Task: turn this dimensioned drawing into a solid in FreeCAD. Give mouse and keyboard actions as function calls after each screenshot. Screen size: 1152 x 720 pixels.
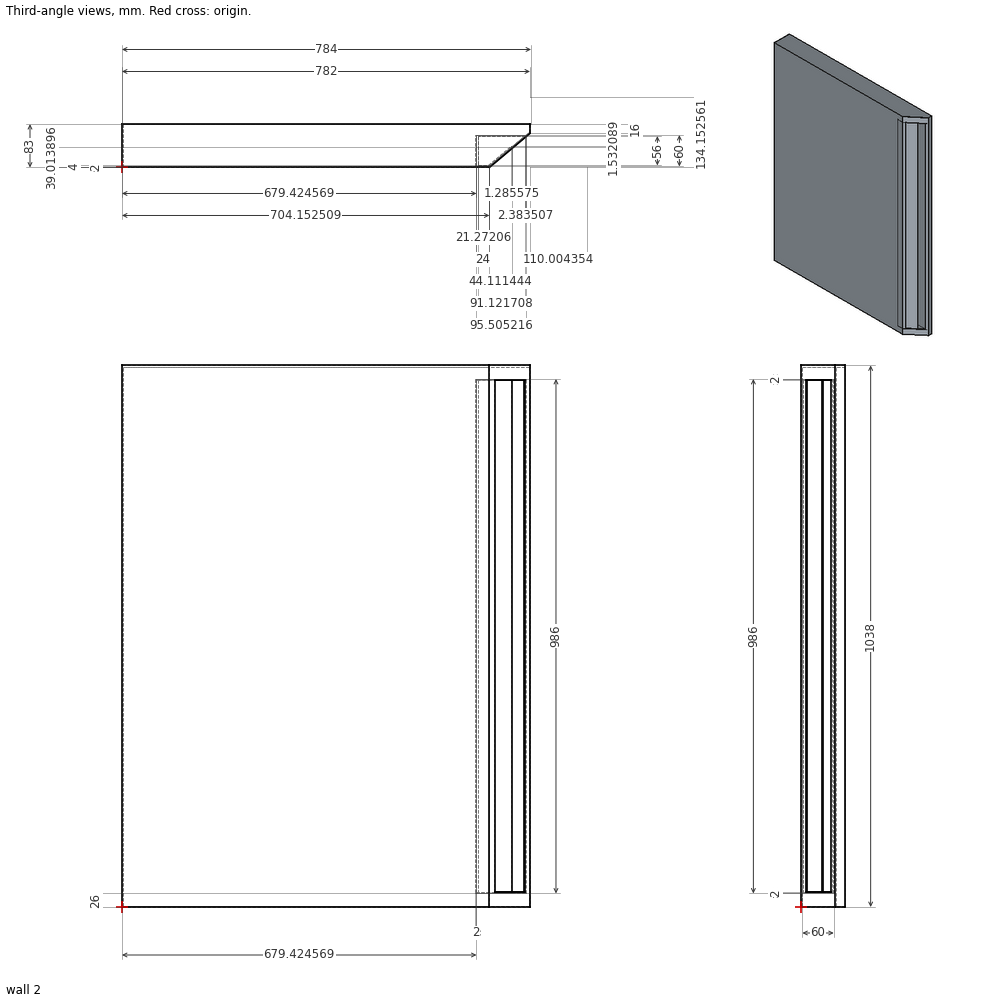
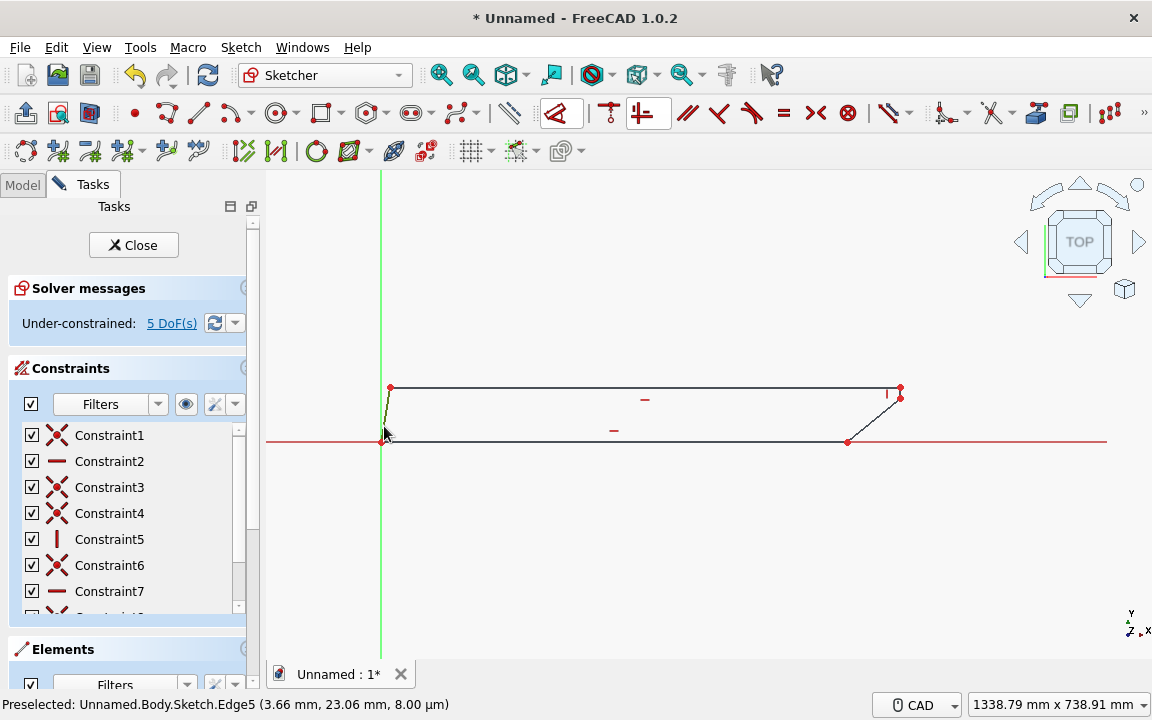
click(666, 114)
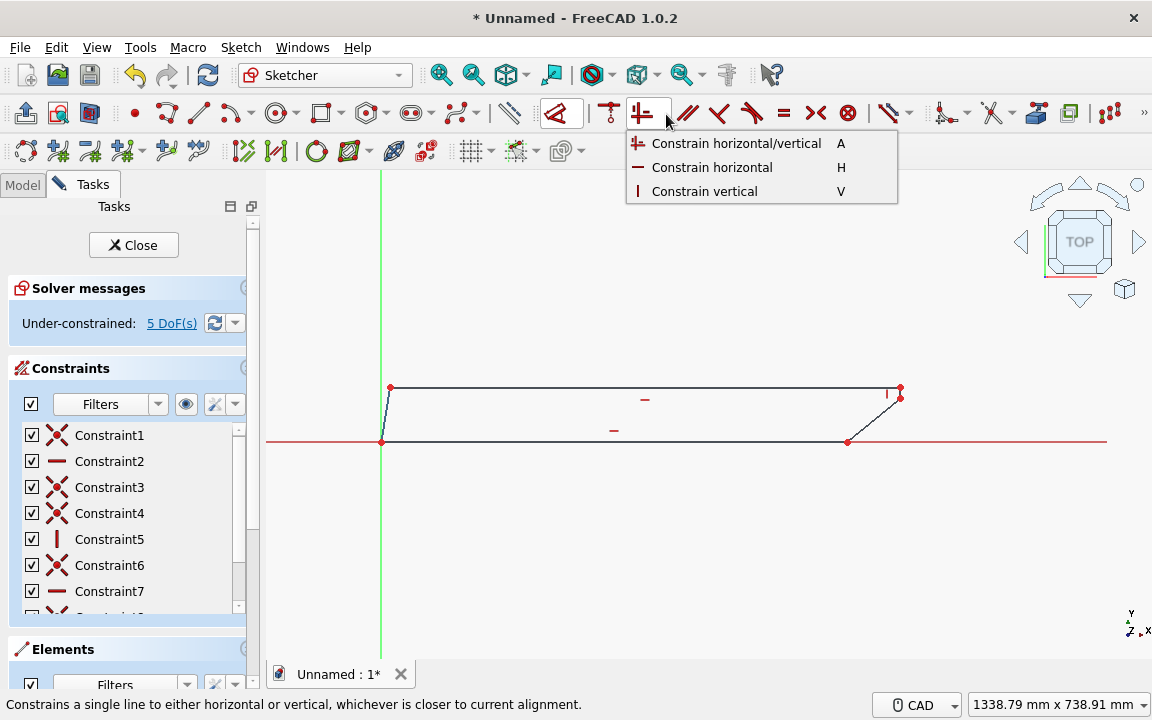
click(762, 191)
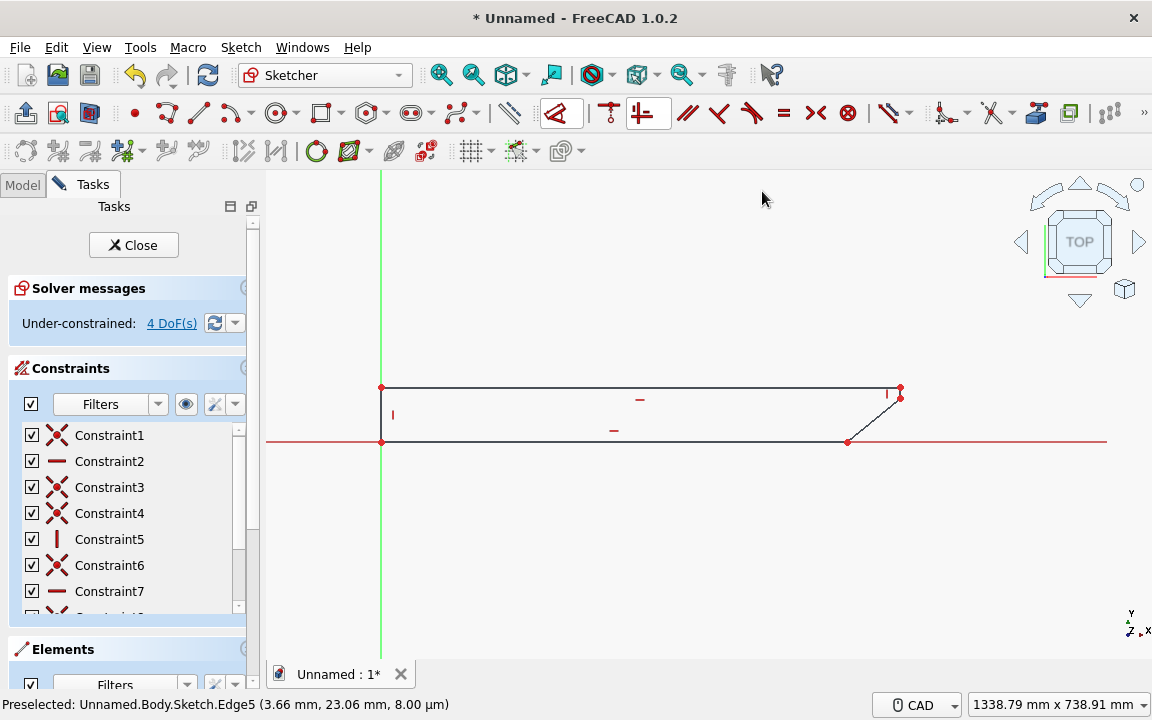
click(556, 114)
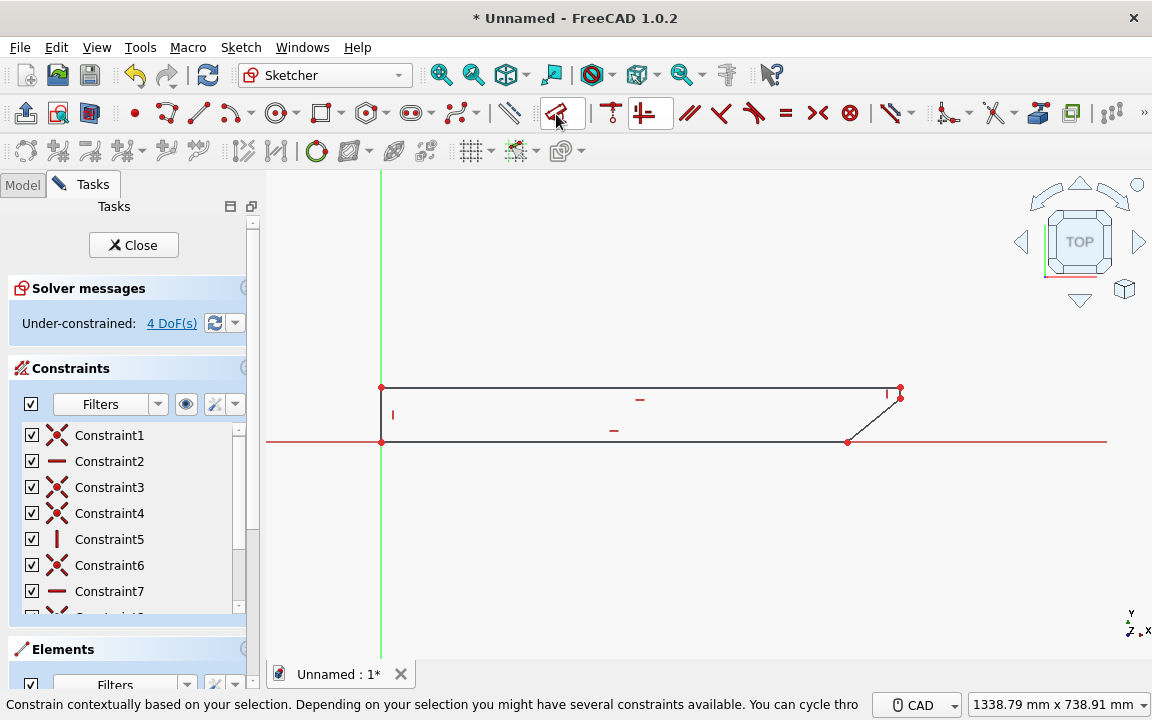
scroll(900, 393, up, 7)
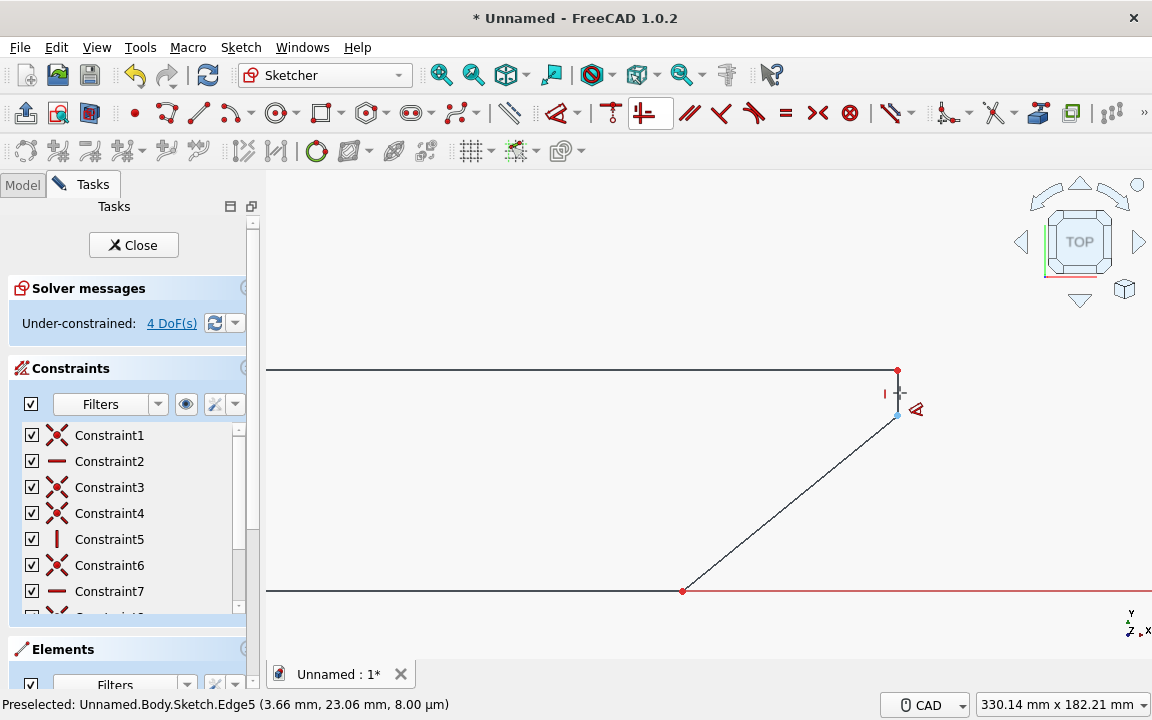
click(898, 393)
click(932, 393)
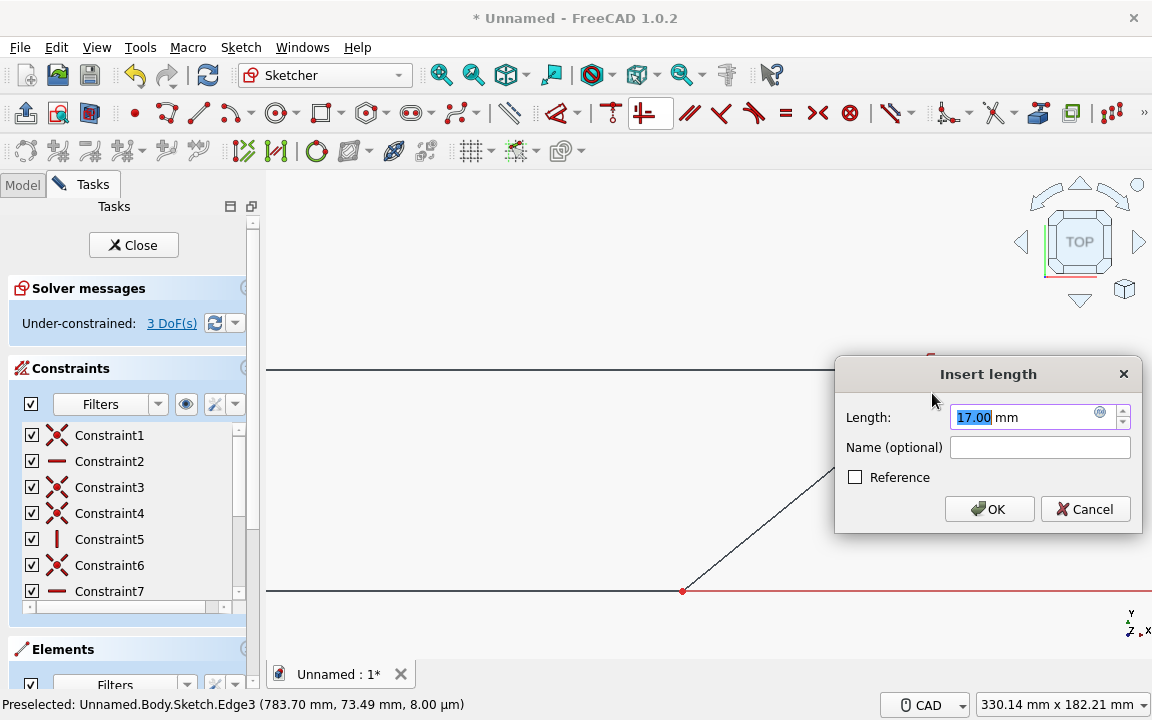
text(16)
key(Return)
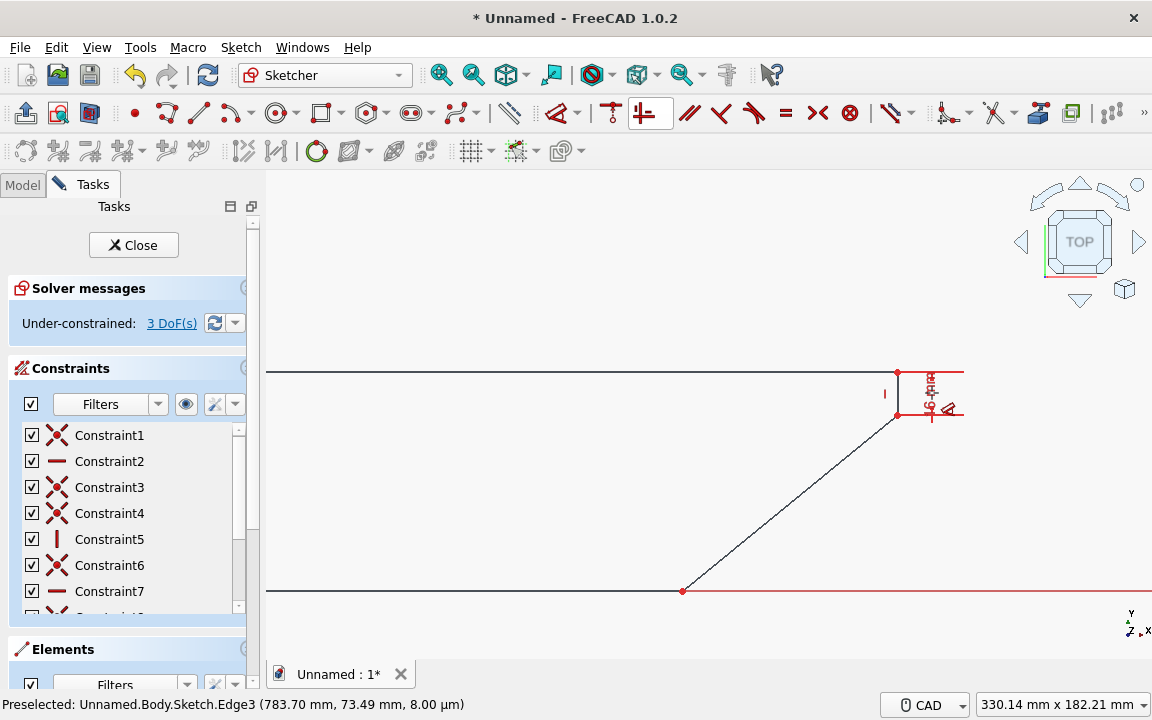
scroll(900, 393, down, 7)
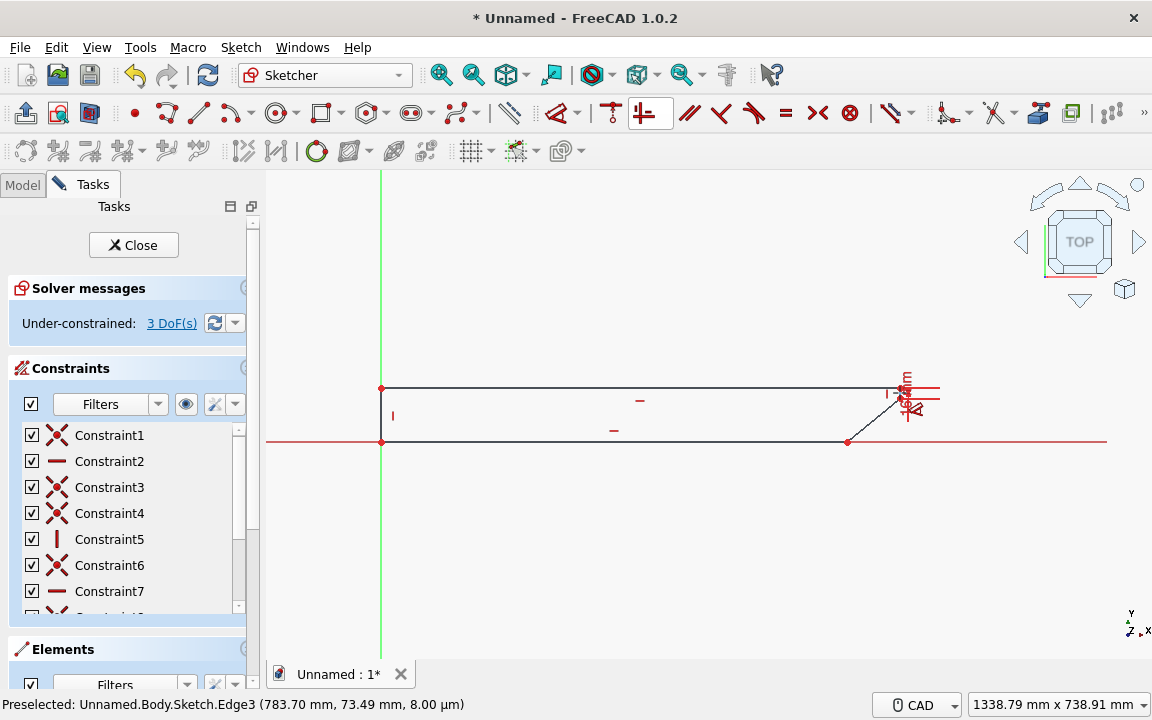
click(381, 404)
click(347, 415)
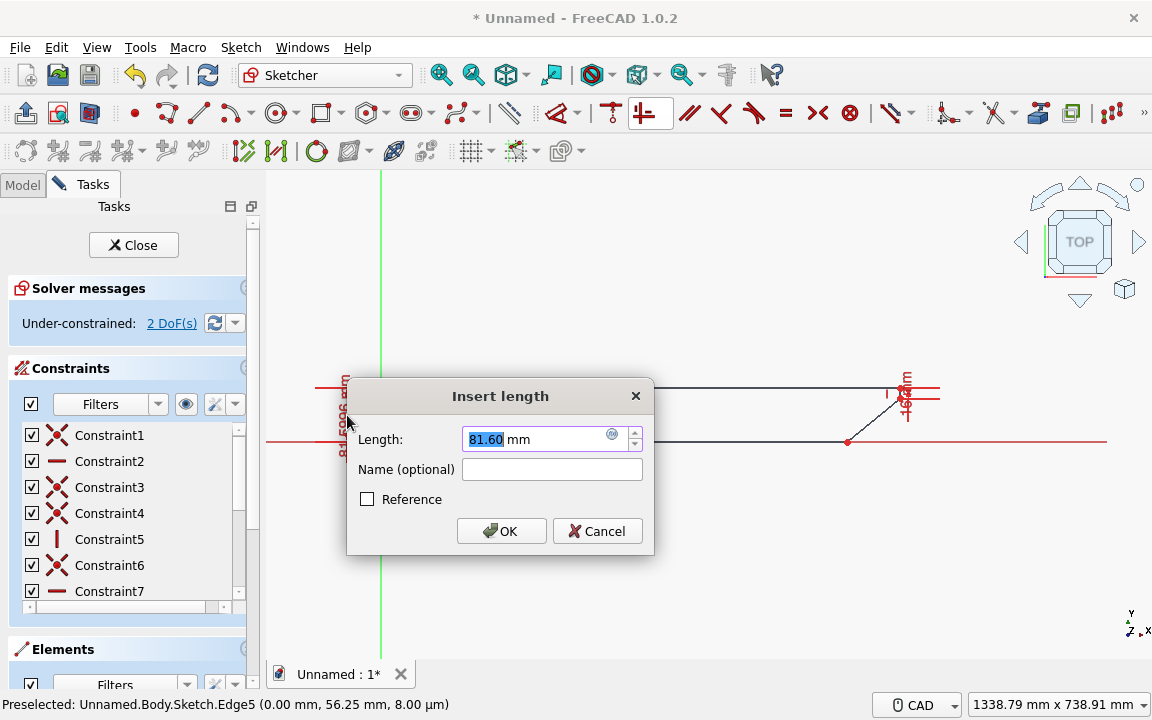
text(83)
key(Return)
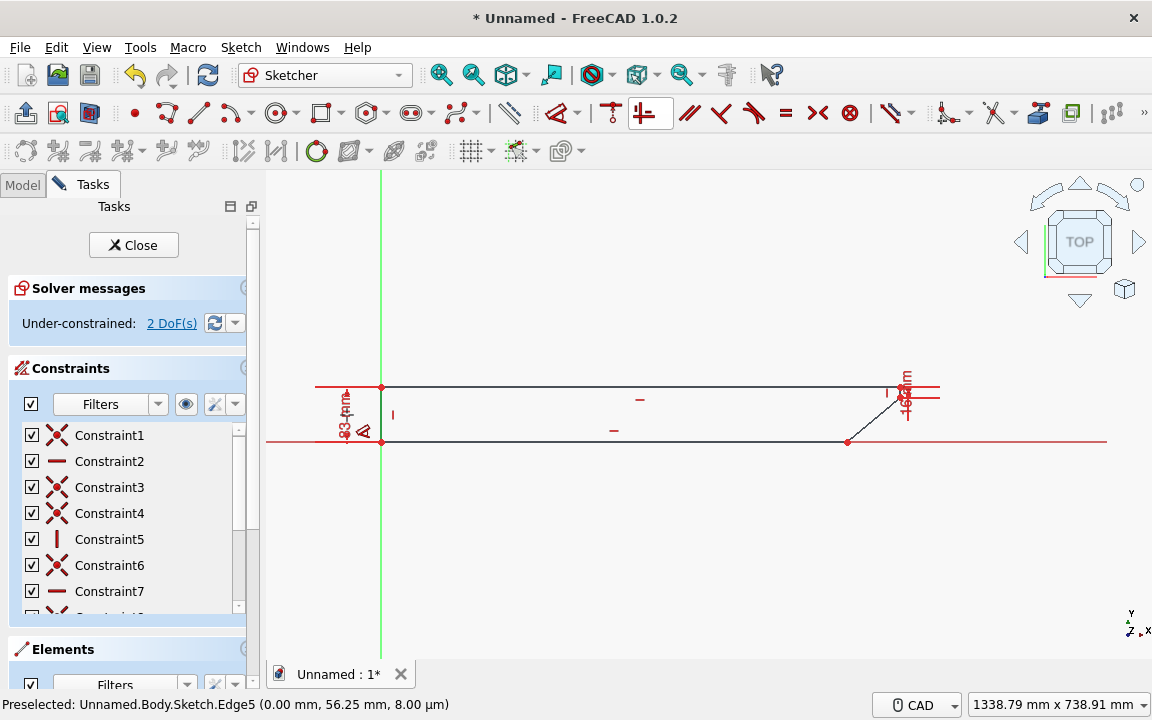
click(744, 387)
click(641, 353)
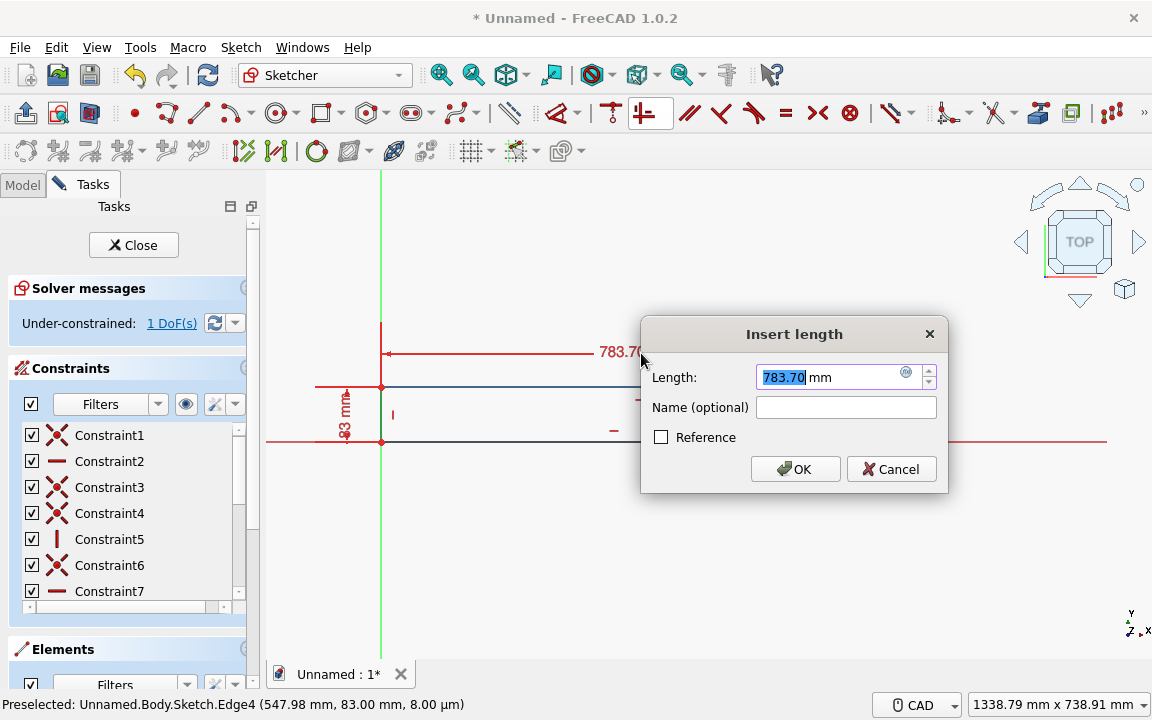
text(784)
key(Return)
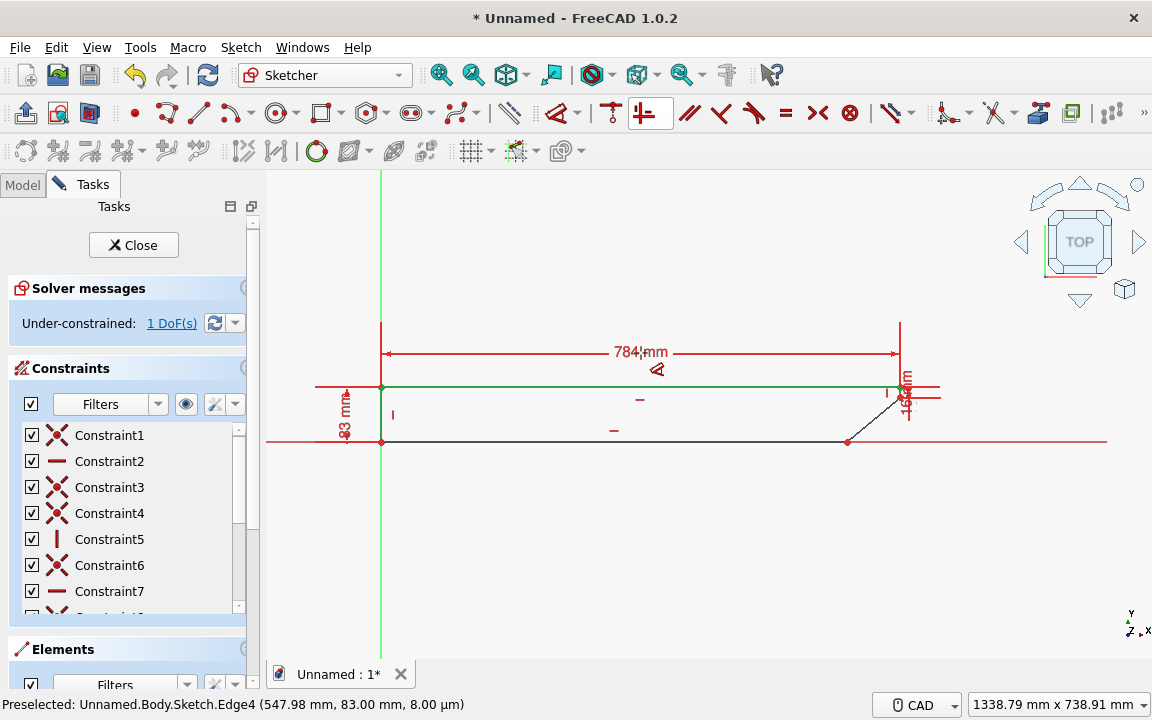
click(521, 442)
click(614, 476)